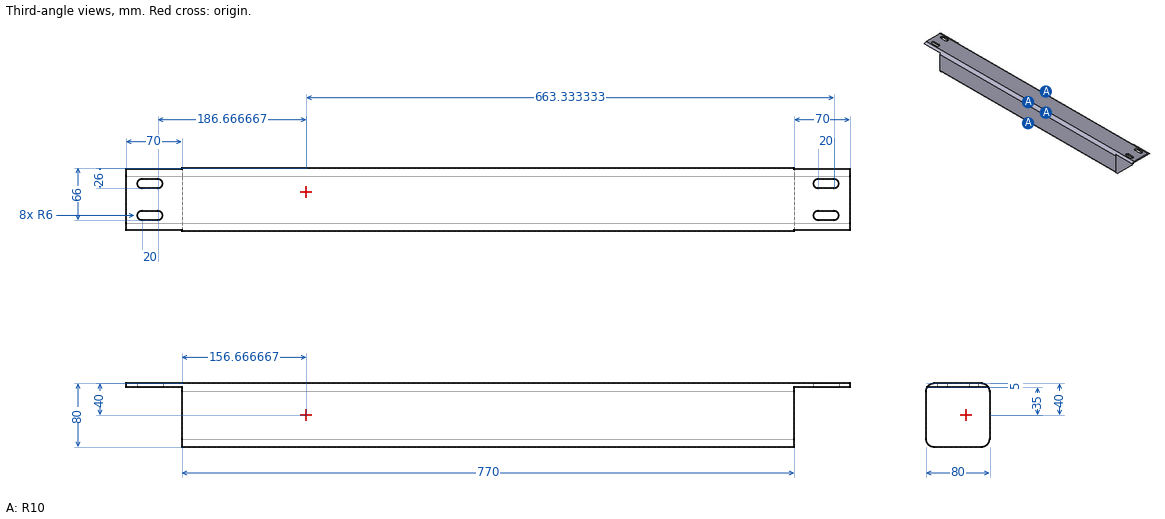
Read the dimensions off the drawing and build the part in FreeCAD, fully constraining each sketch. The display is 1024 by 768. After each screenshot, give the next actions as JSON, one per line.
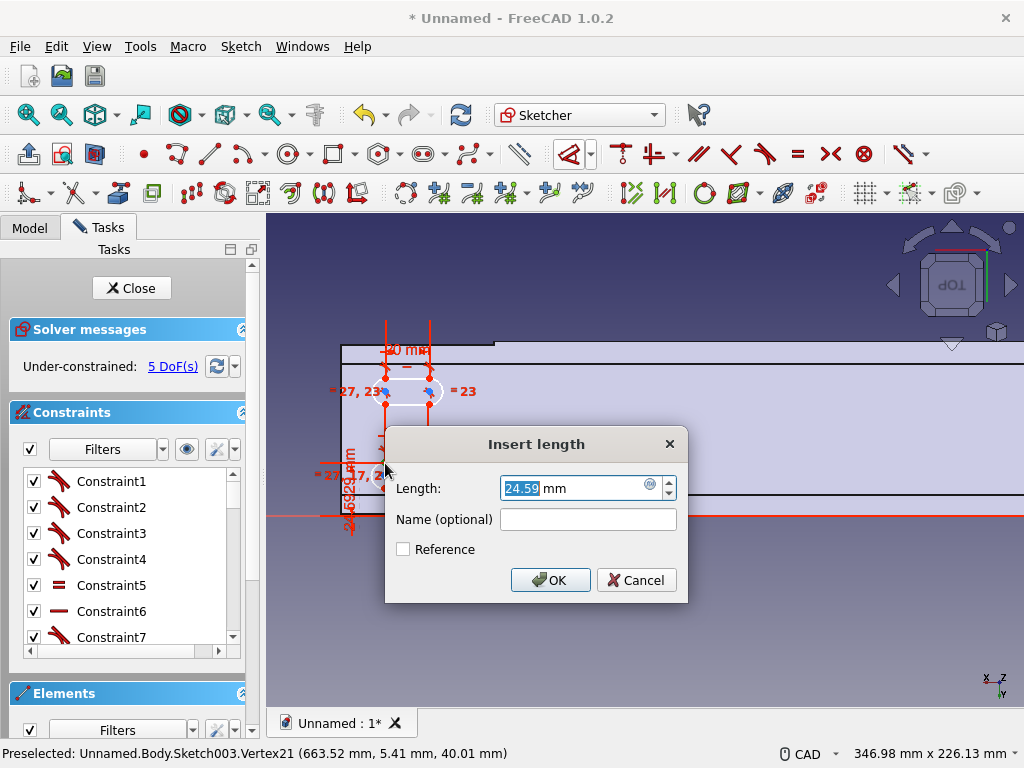
{"action": "type", "text": "26"}
{"action": "key", "text": "Return"}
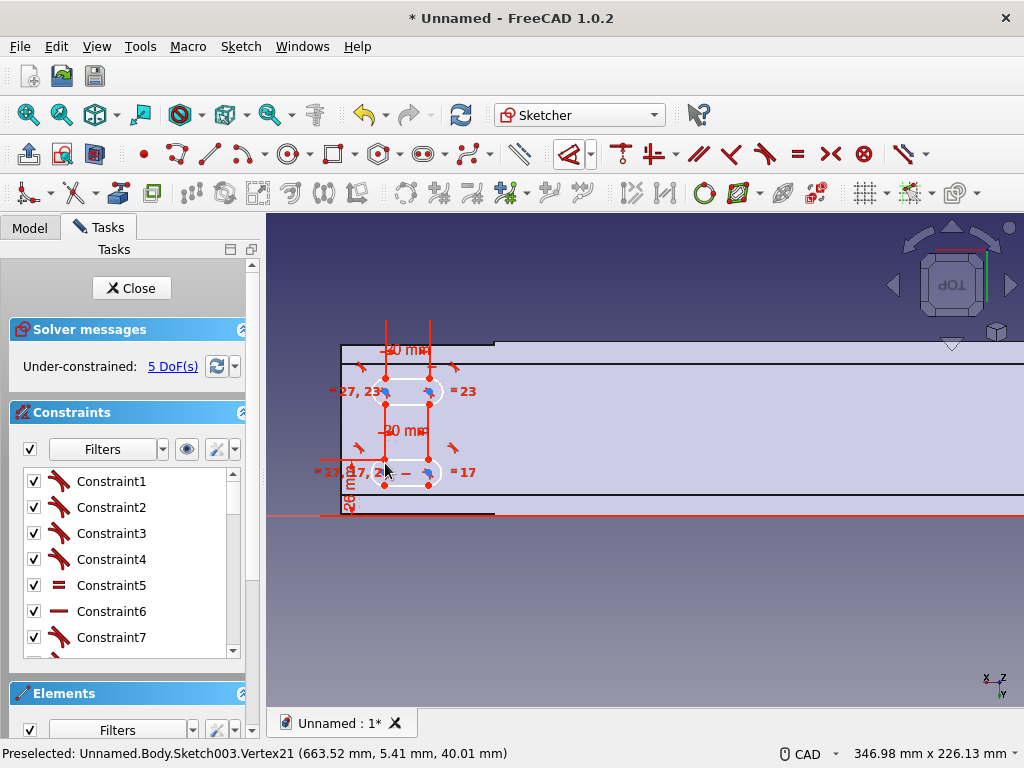
{"action": "left_click", "coordinate": [386, 379]}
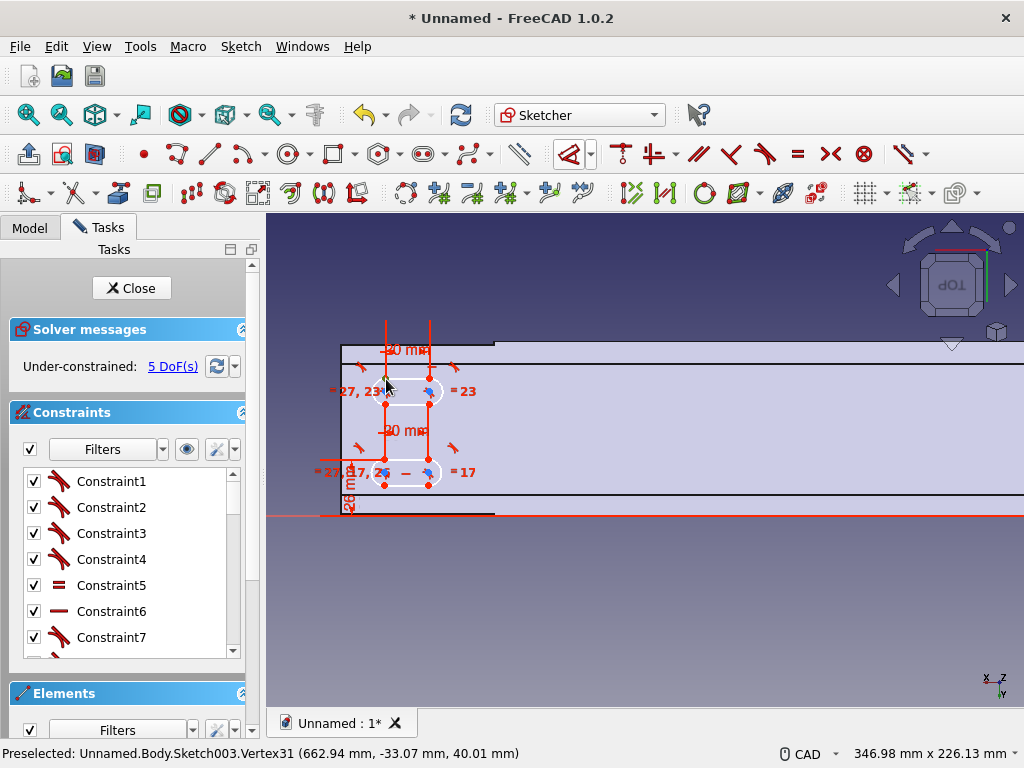
{"action": "key", "text": "i"}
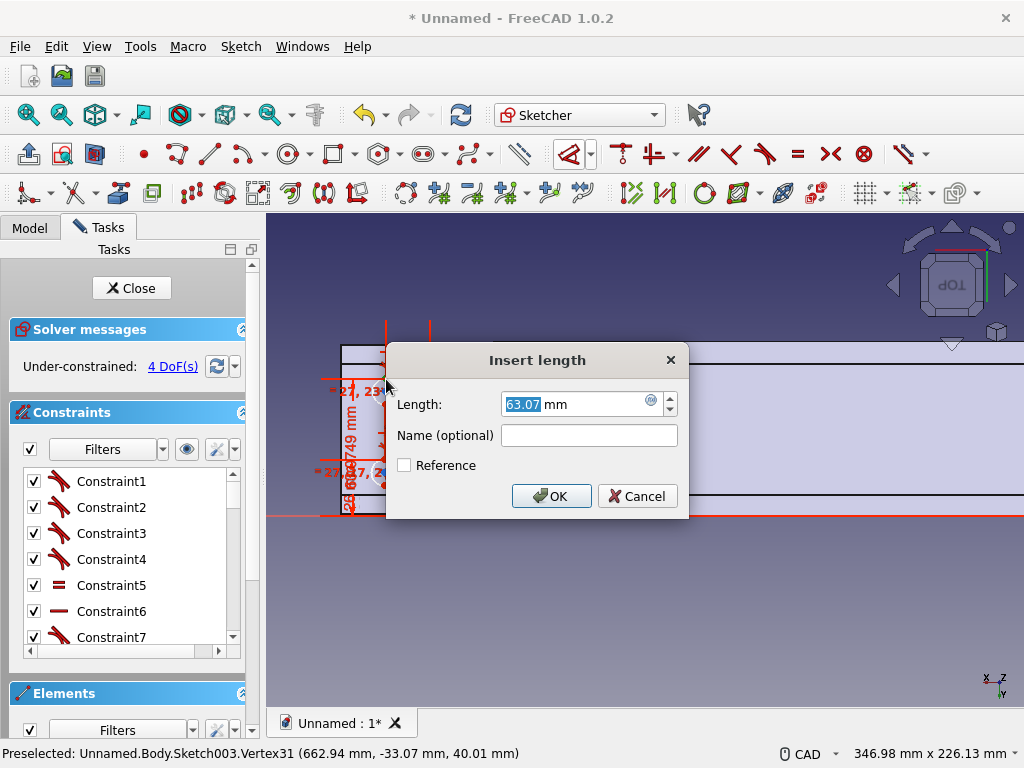
{"action": "type", "text": "66"}
{"action": "key", "text": "Return"}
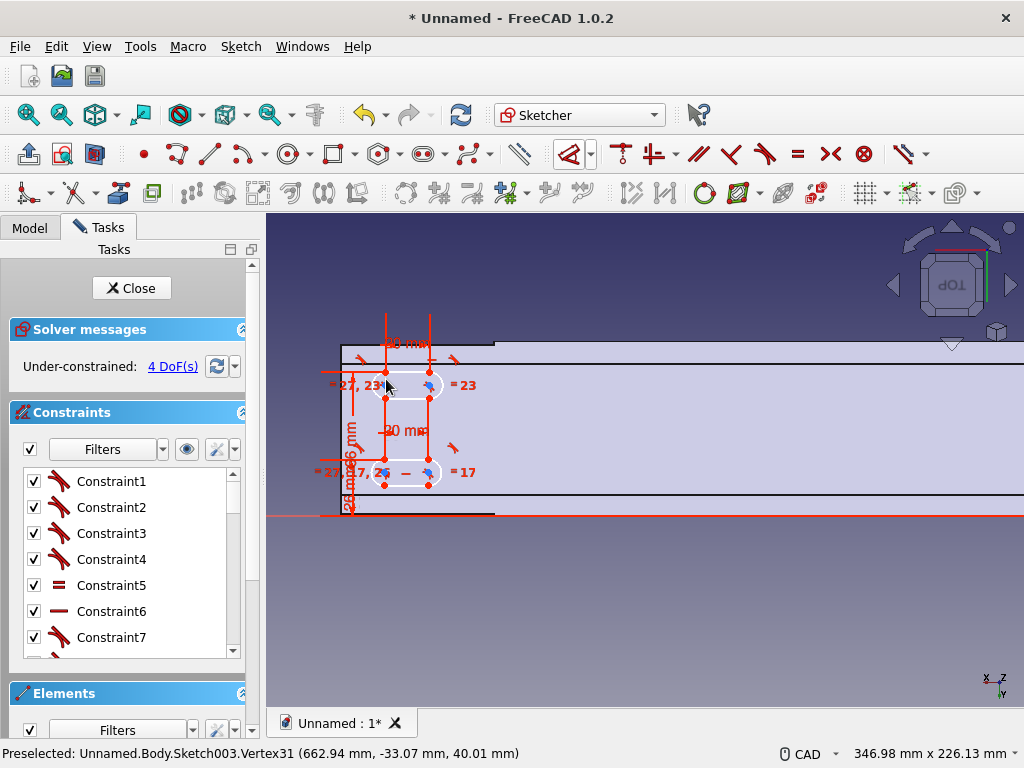
{"action": "scroll", "coordinate": [385, 464], "scroll_direction": "down", "scroll_amount": 8}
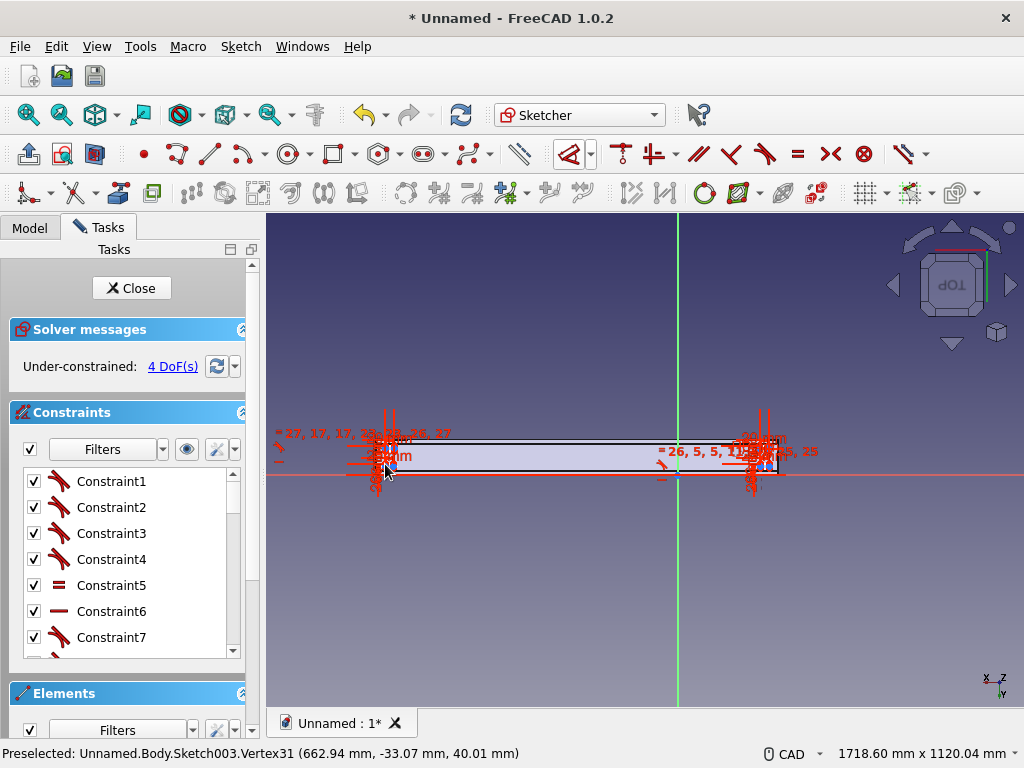
{"action": "scroll", "coordinate": [760, 446], "scroll_direction": "up", "scroll_amount": 8}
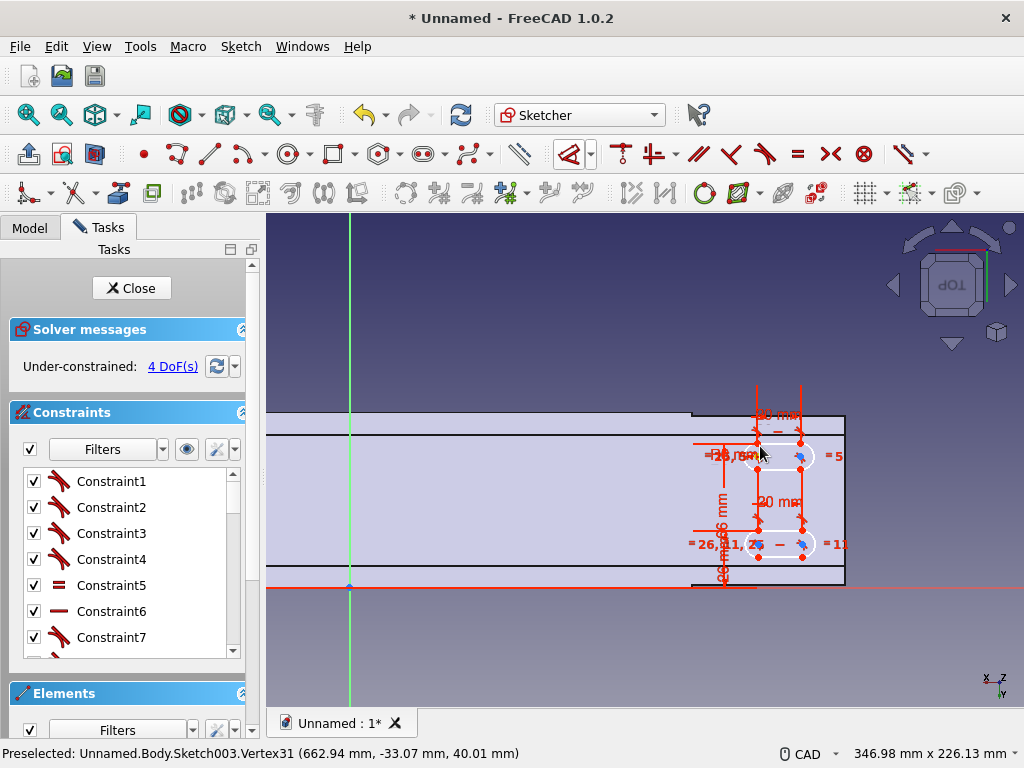
{"action": "left_click", "coordinate": [757, 444]}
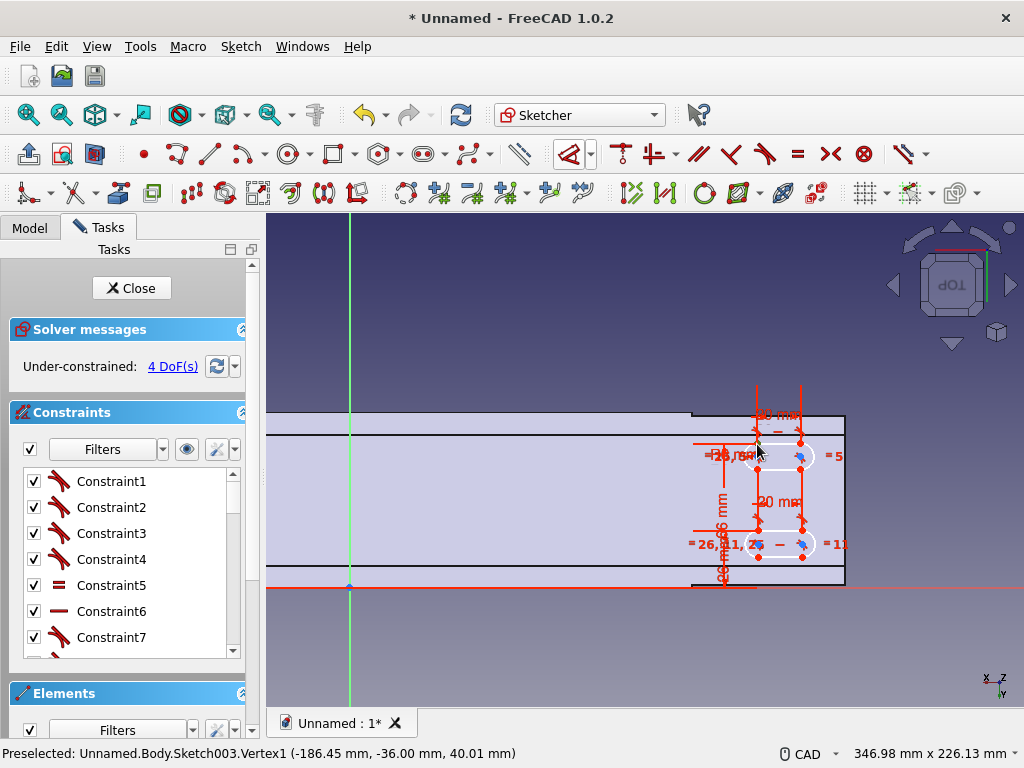
{"action": "left_click", "coordinate": [590, 154]}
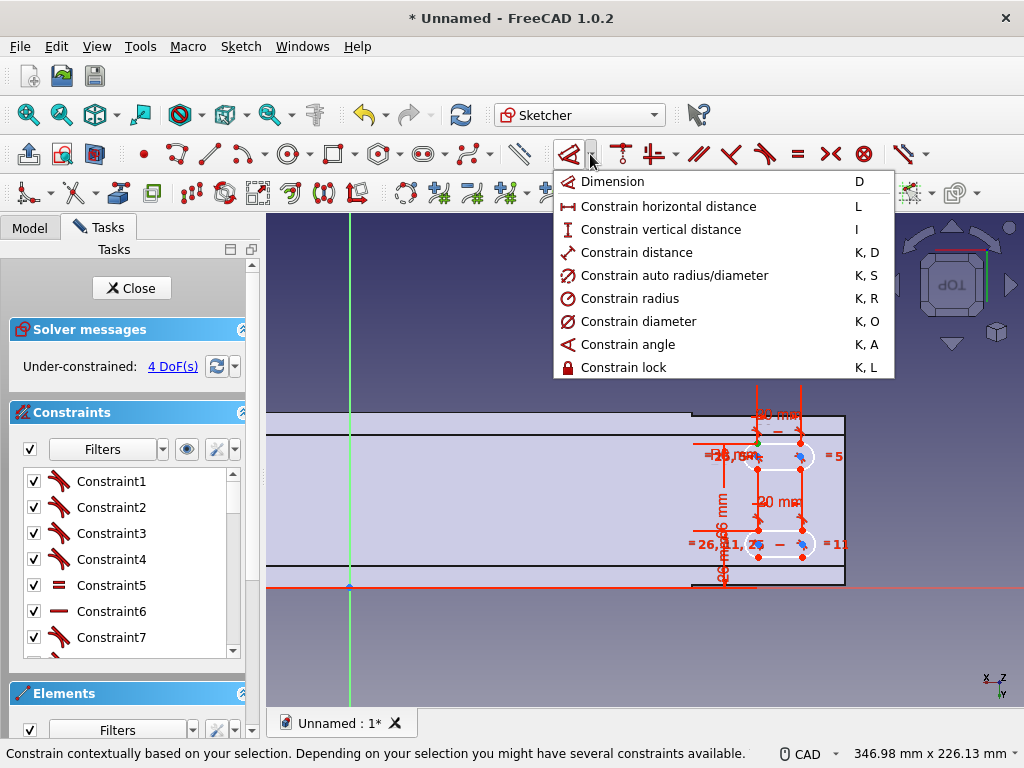
{"action": "left_click", "coordinate": [724, 206]}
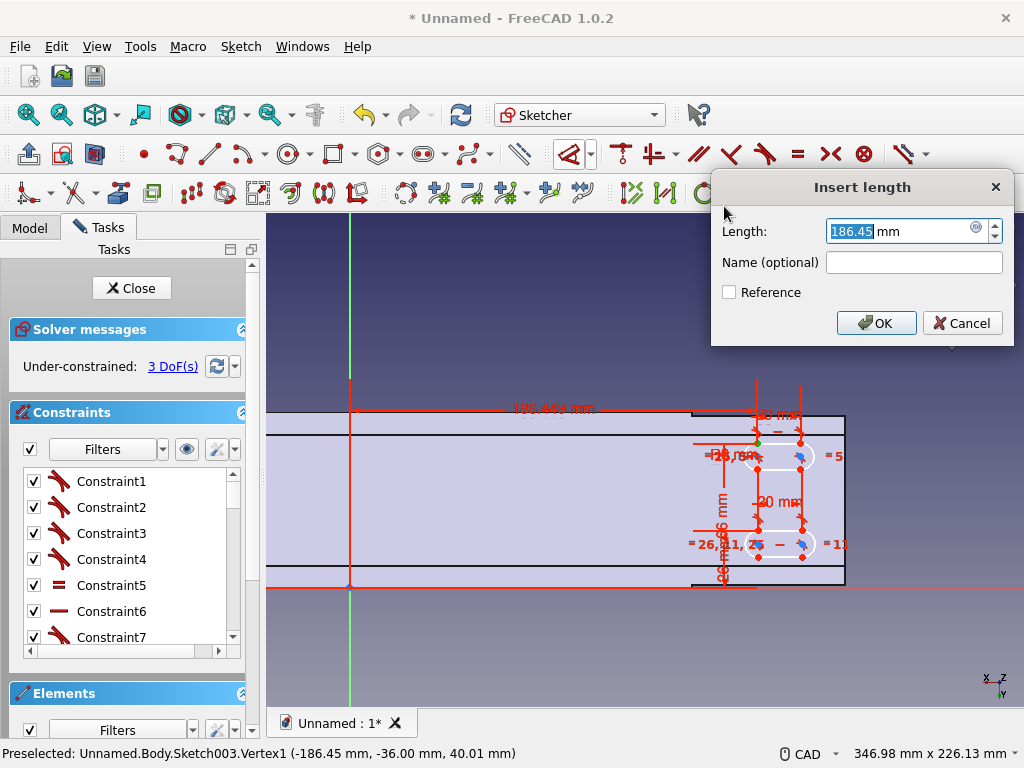
{"action": "type", "text": "186.666667"}
{"action": "key", "text": "Return"}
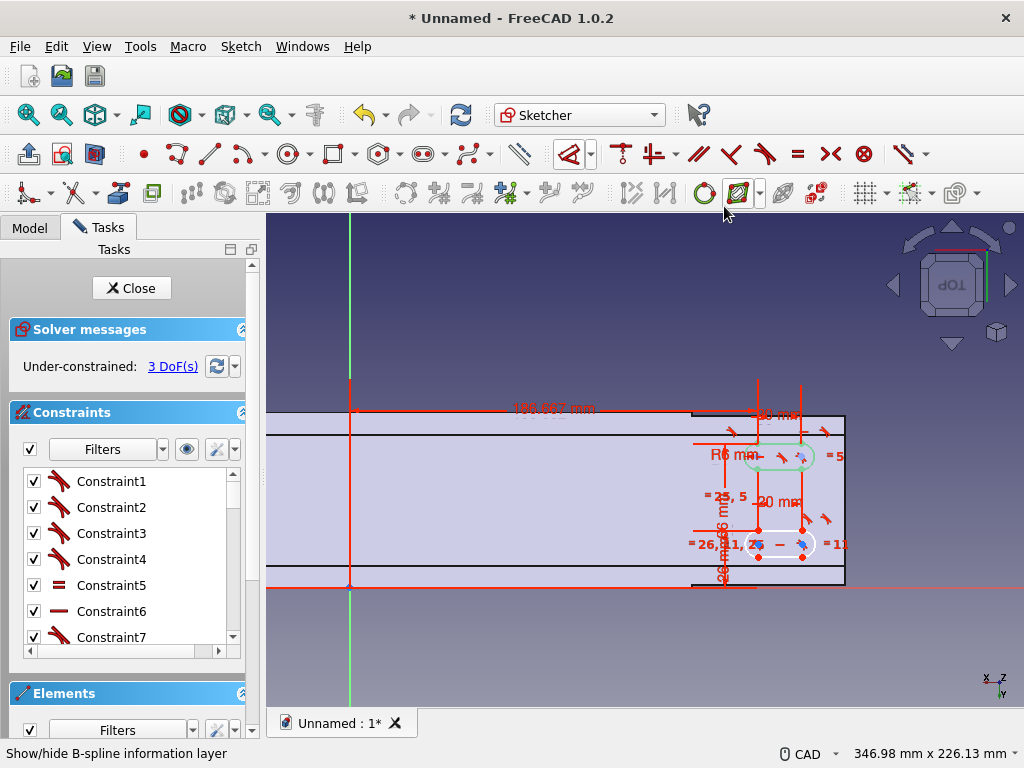
{"action": "left_click", "coordinate": [758, 531]}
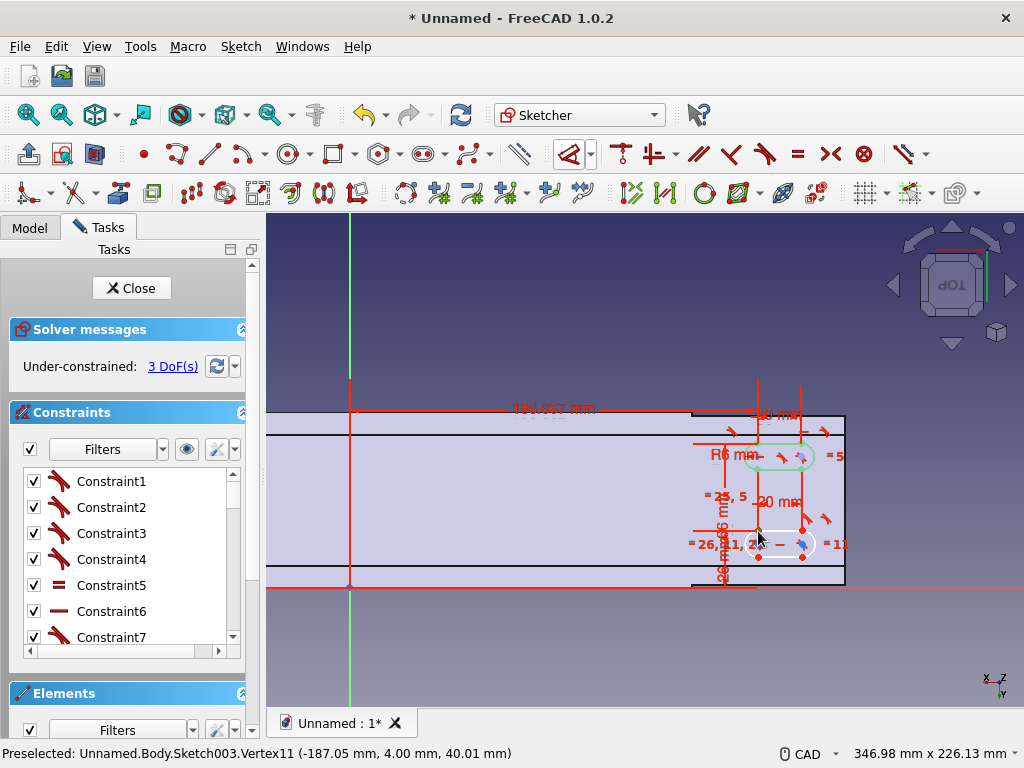
{"action": "key", "text": "l"}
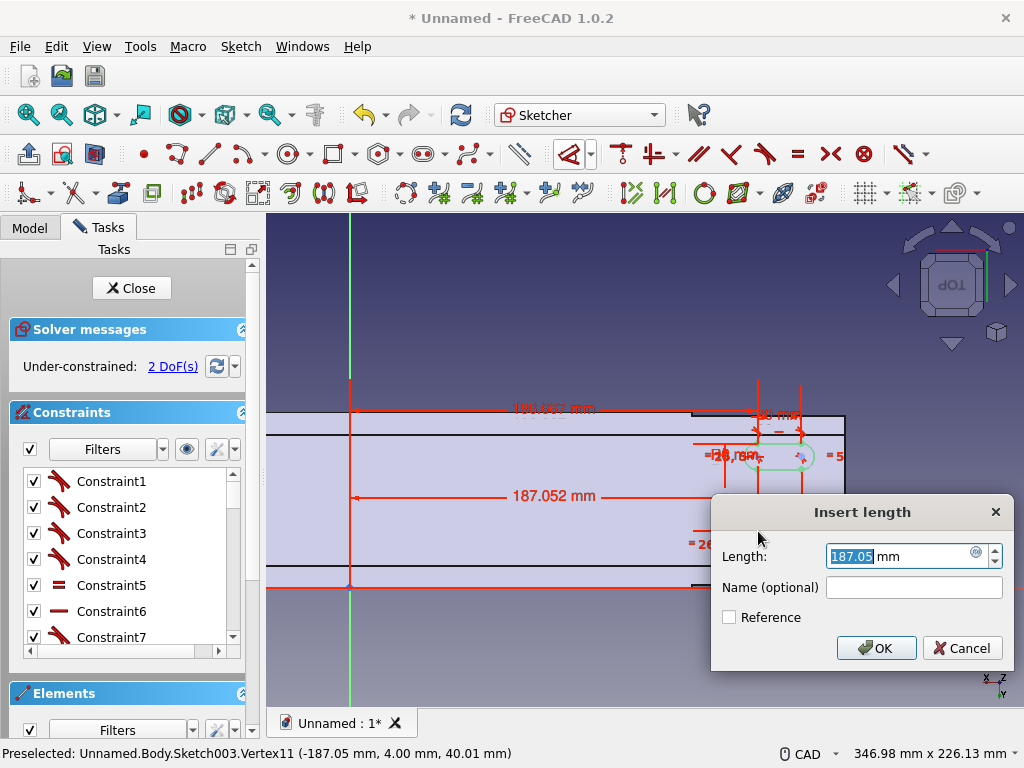
{"action": "type", "text": "186.666667"}
{"action": "key", "text": "Return"}